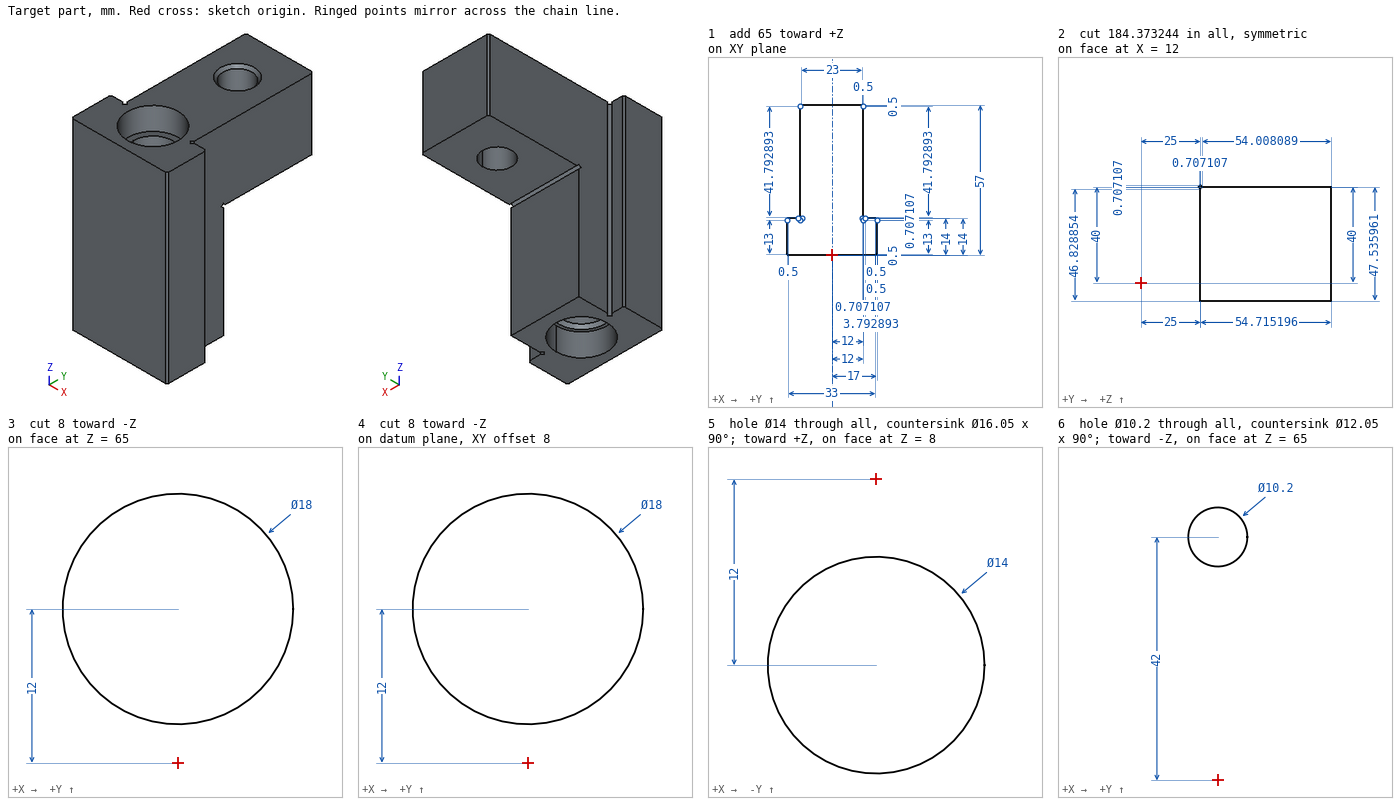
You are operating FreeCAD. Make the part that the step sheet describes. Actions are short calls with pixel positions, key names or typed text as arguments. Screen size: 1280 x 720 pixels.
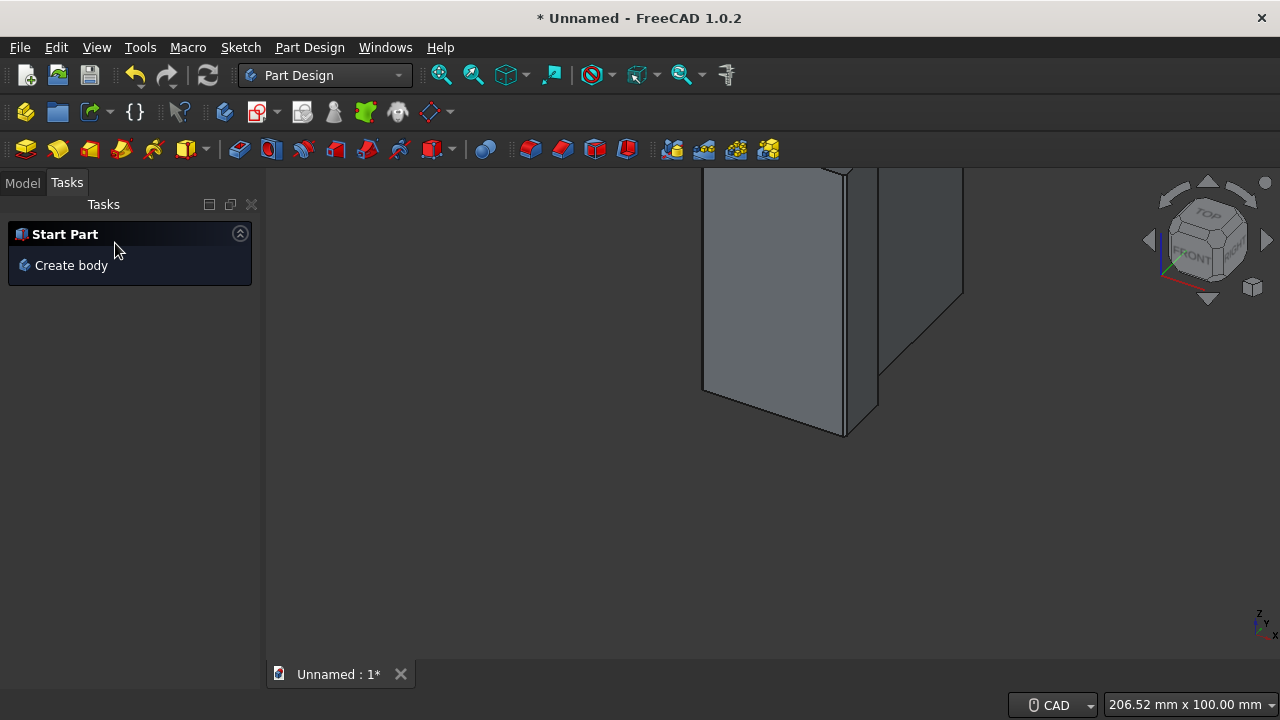
key(v)
key(f)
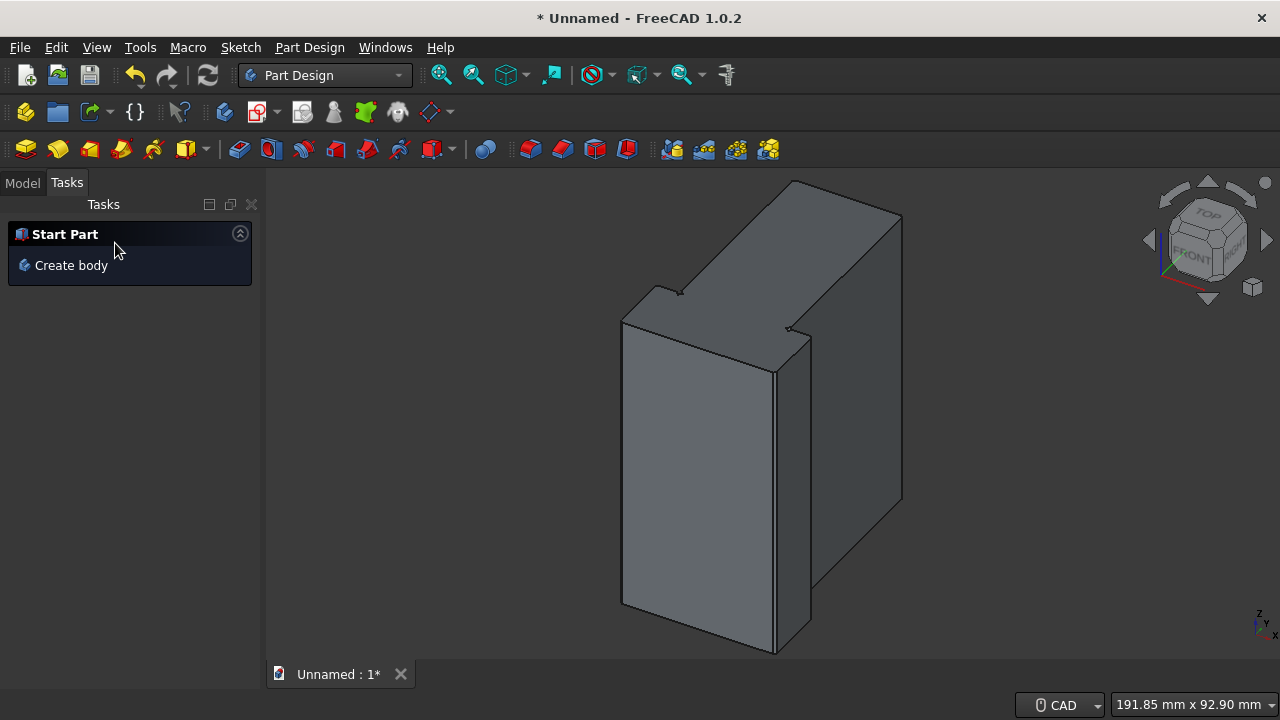
click(847, 372)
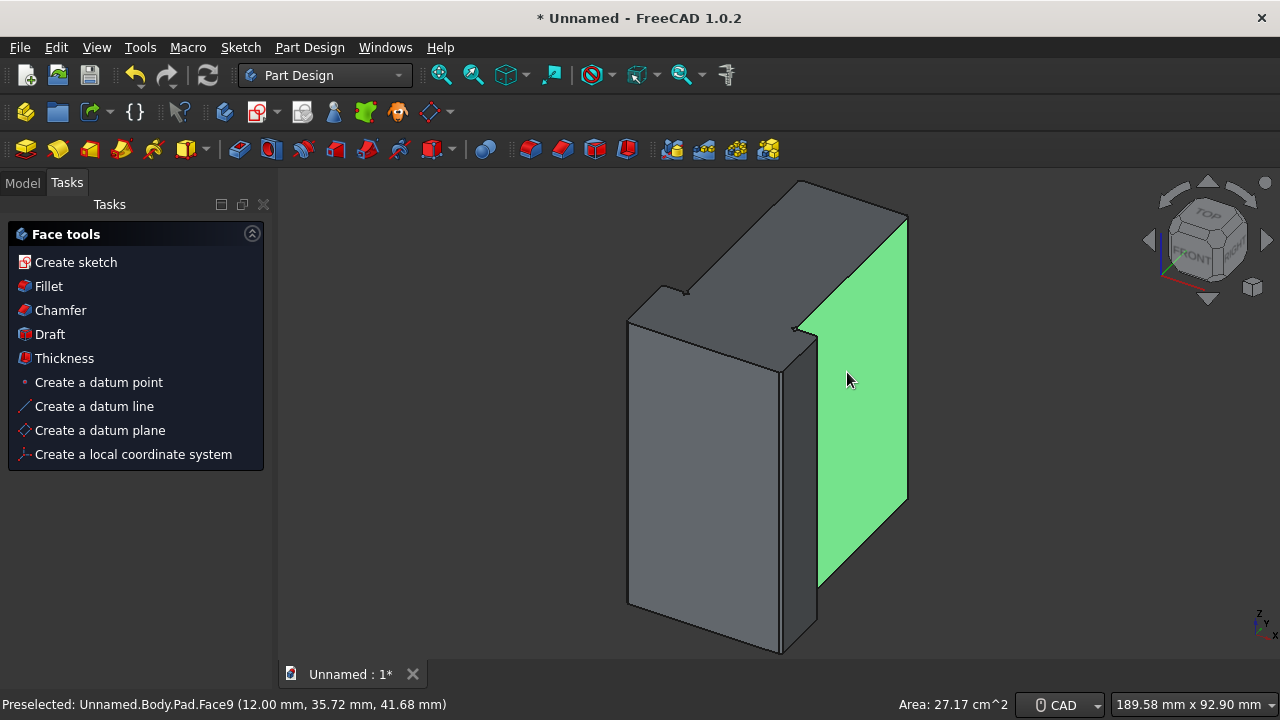
click(258, 112)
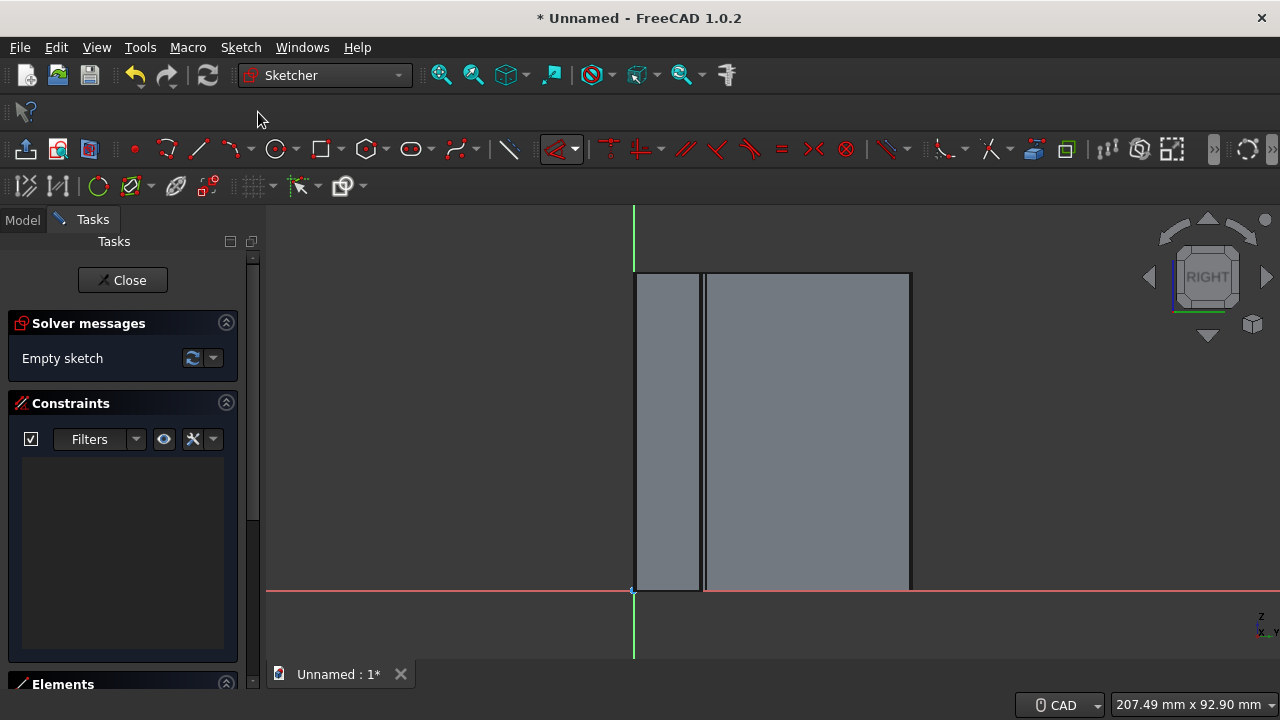
scroll(294, 233, down, 1)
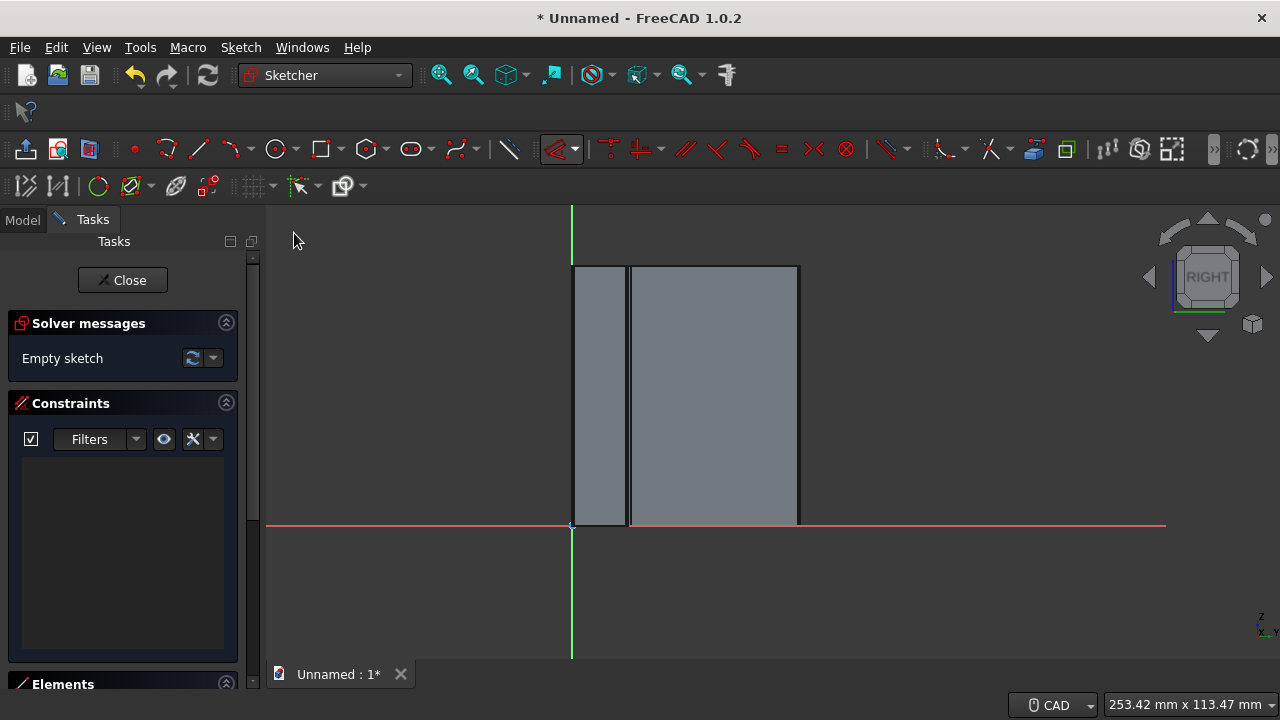
scroll(787, 516, up, 2)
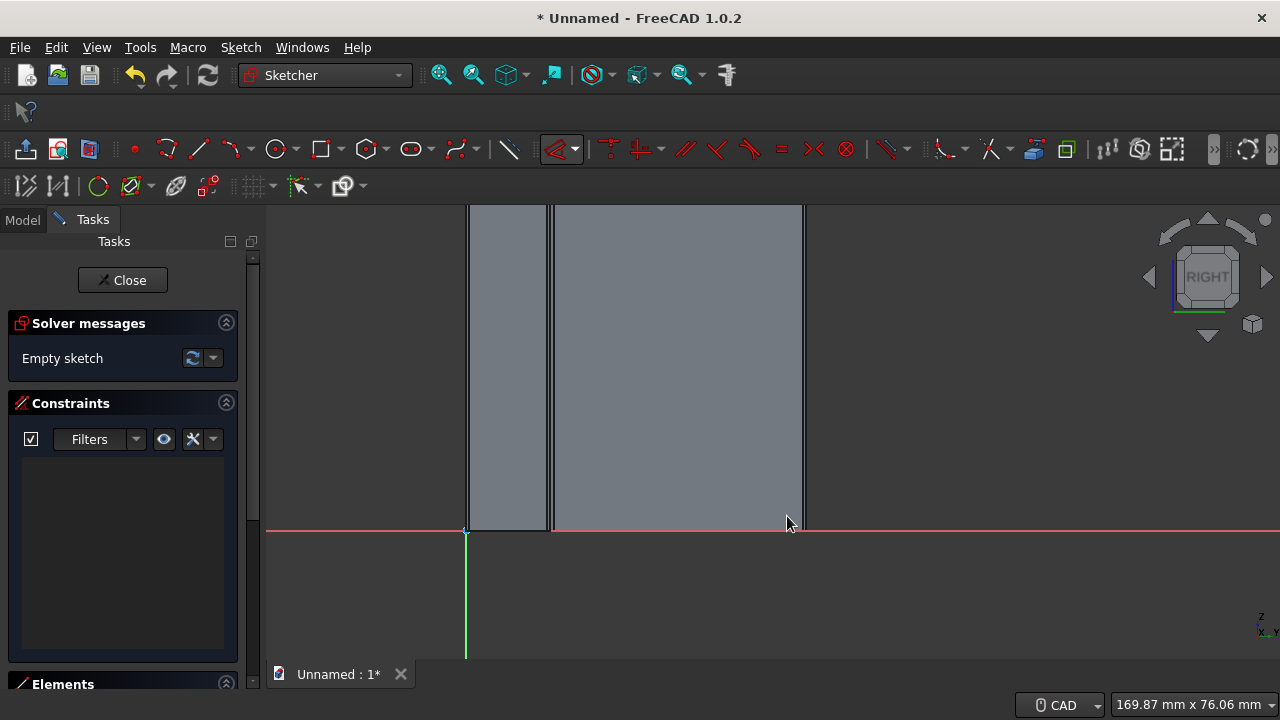
click(168, 150)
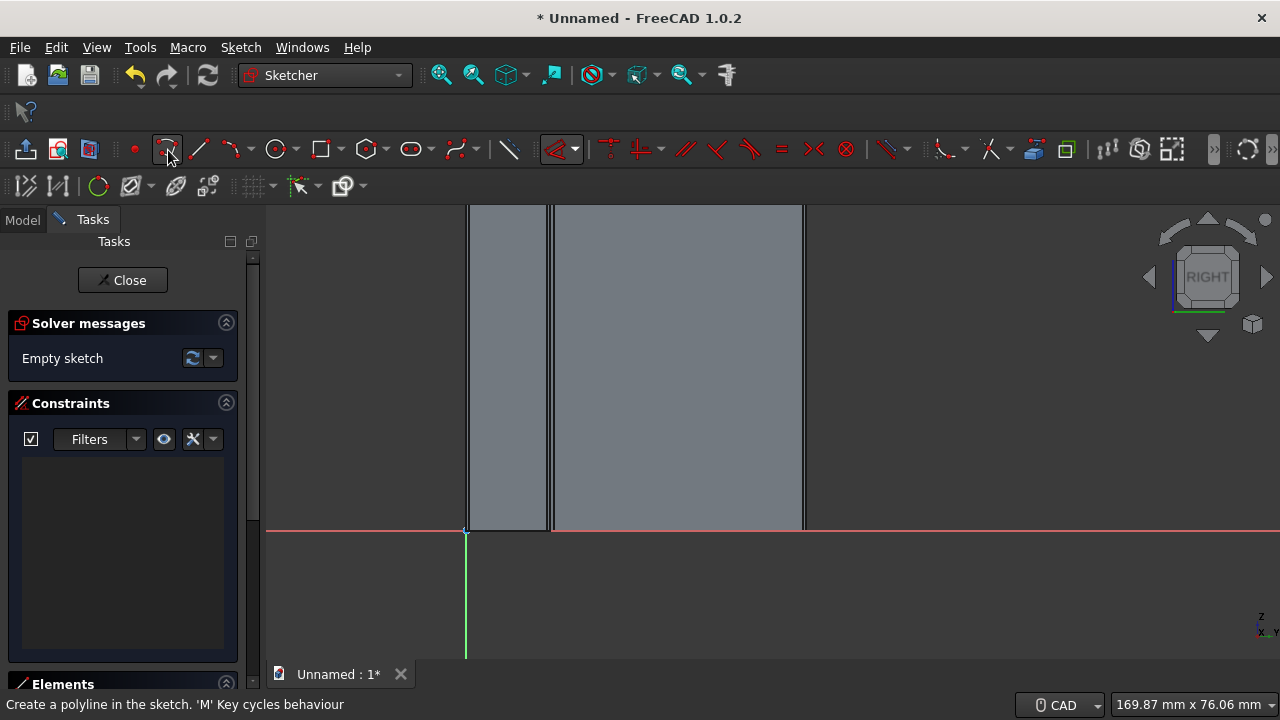
click(615, 576)
click(942, 576)
click(942, 292)
click(620, 292)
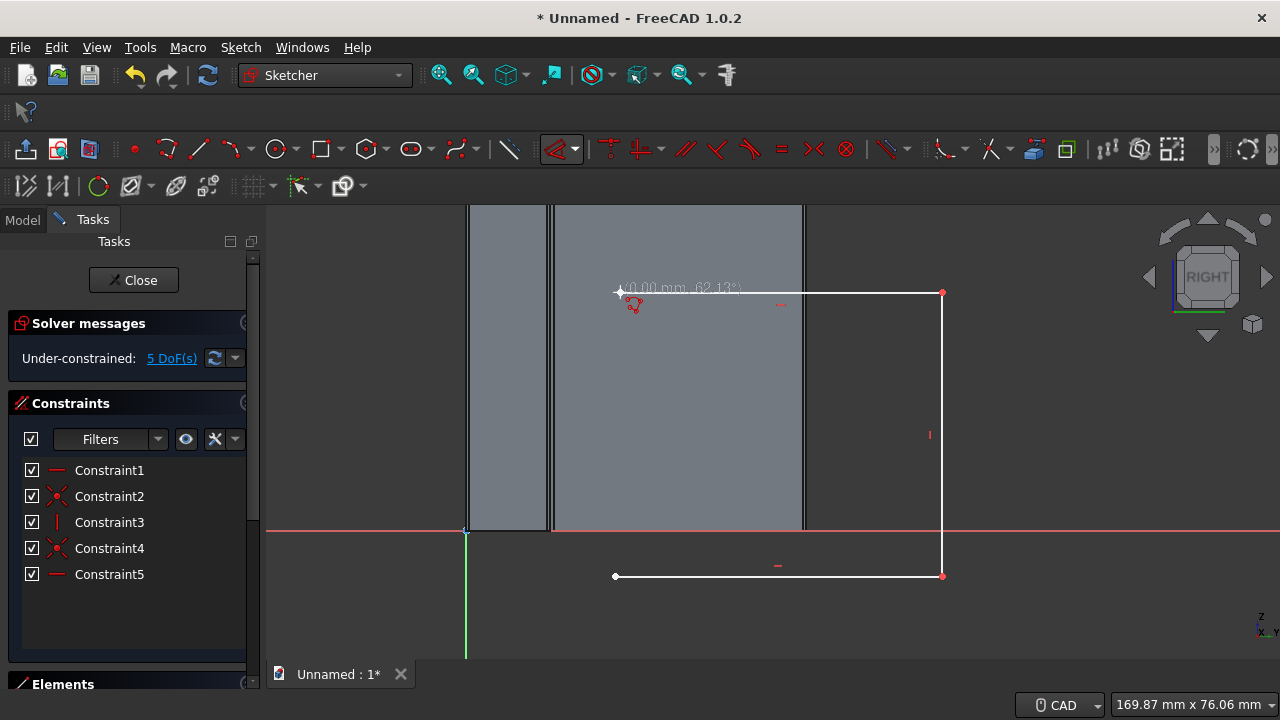
scroll(615, 288, up, 5)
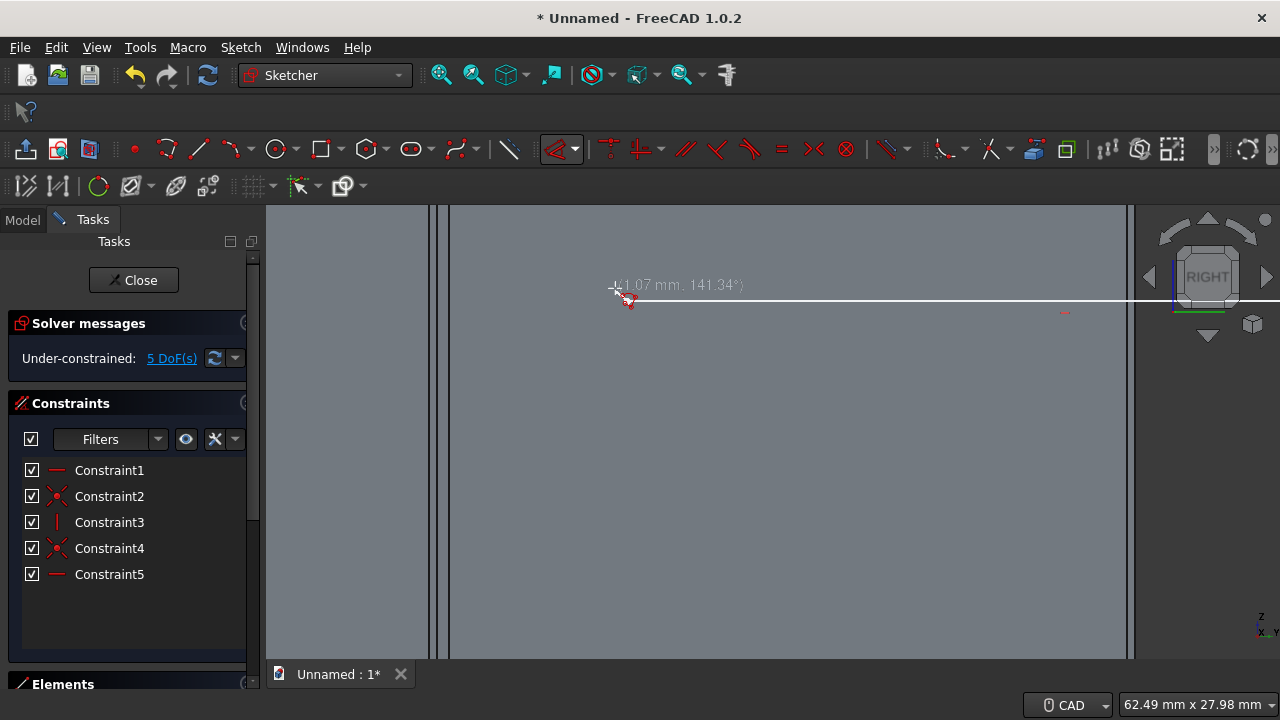
click(616, 286)
click(604, 298)
click(616, 309)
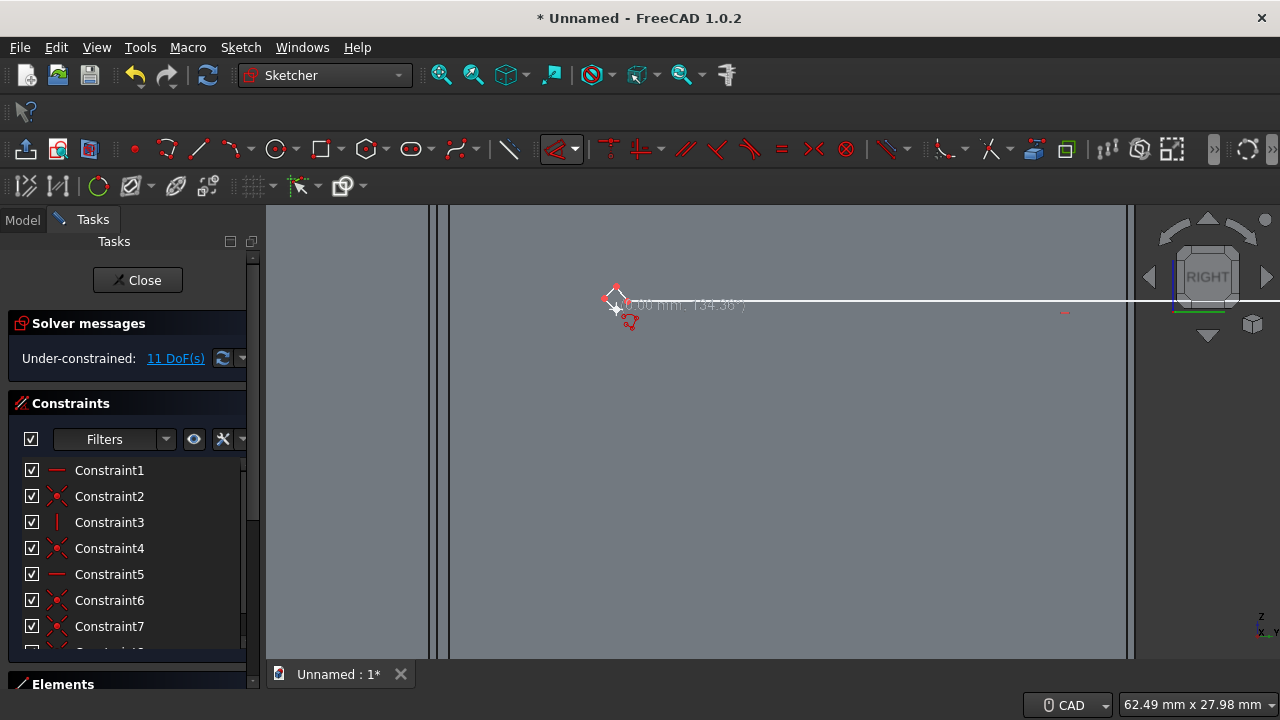
scroll(616, 289, down, 5)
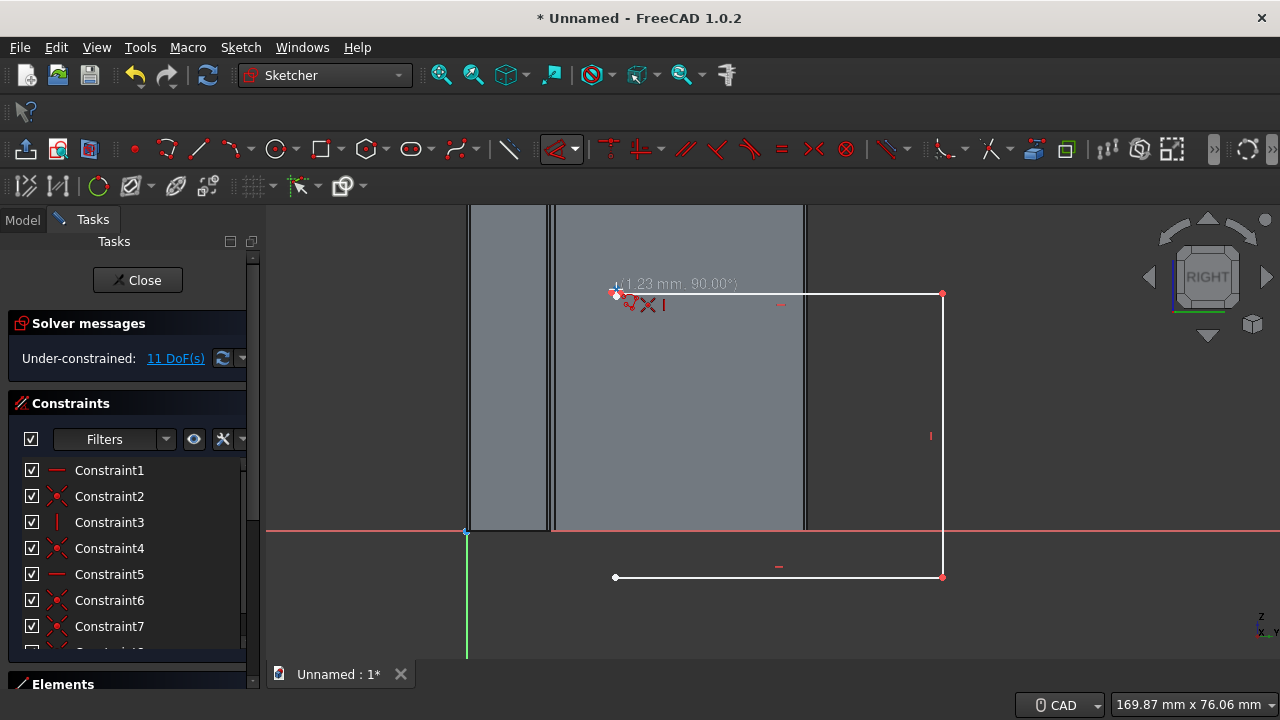
click(616, 578)
key(Escape)
key(Escape)